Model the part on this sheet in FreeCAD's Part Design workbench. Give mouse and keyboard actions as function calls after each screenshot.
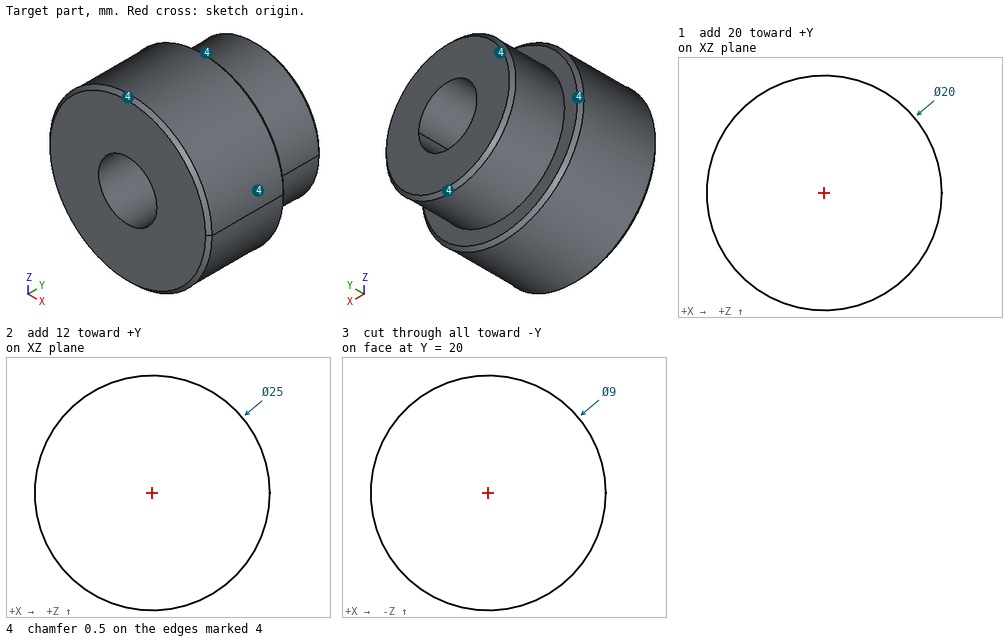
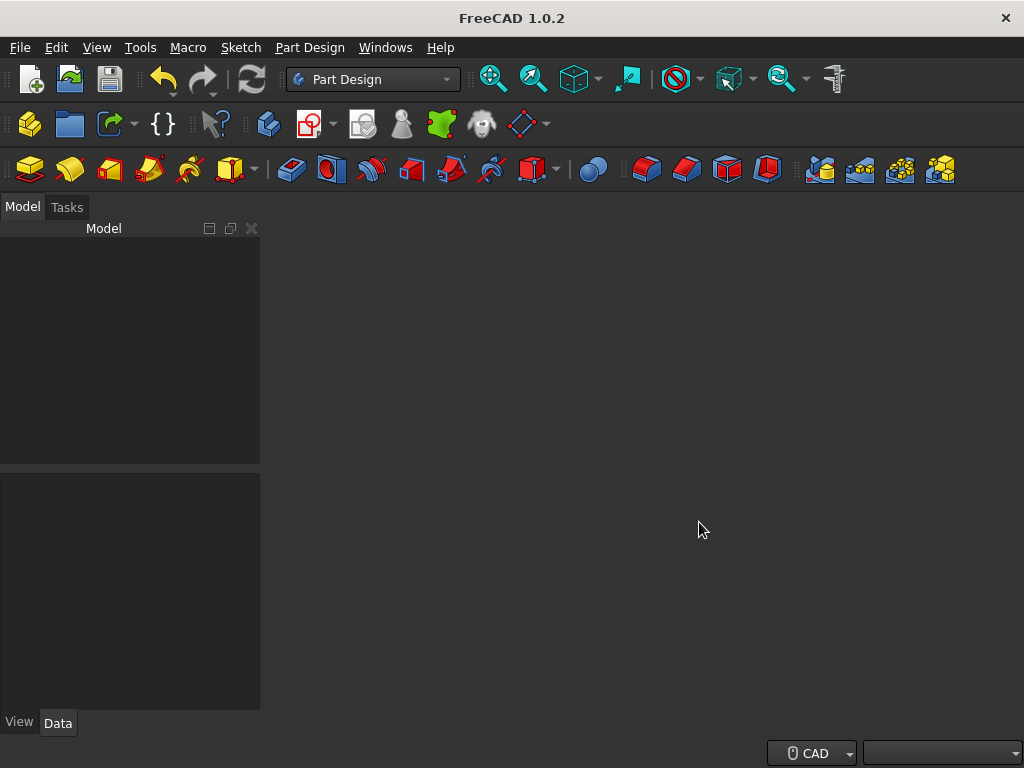
click(30, 80)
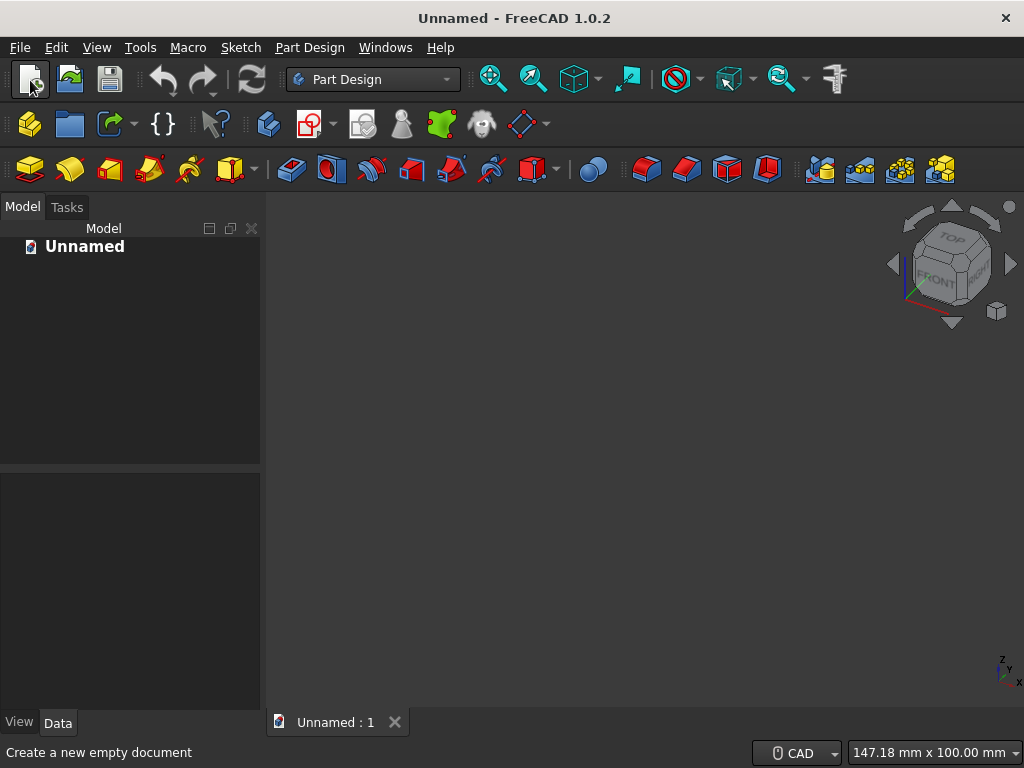
click(310, 124)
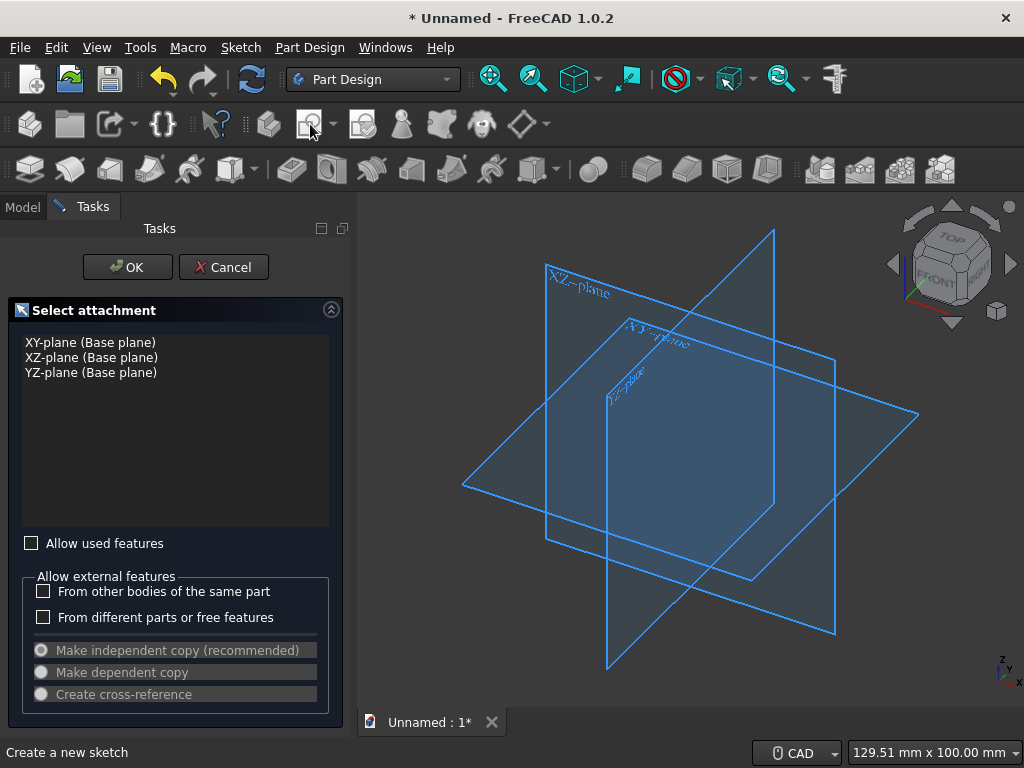
click(82, 358)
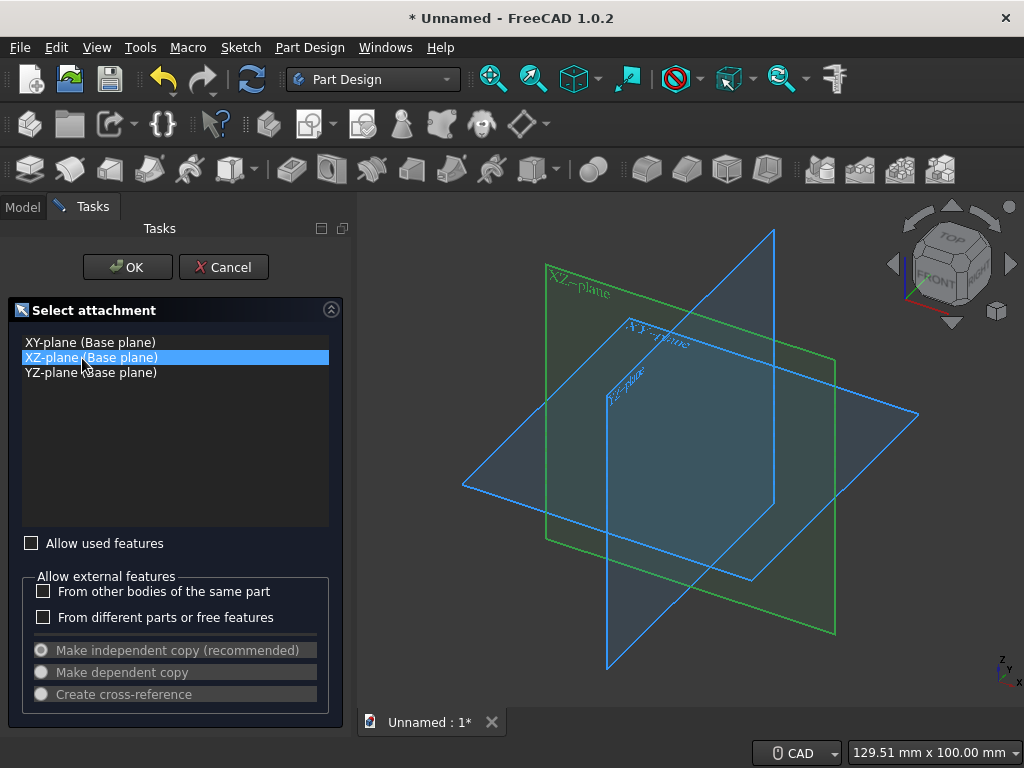
click(128, 267)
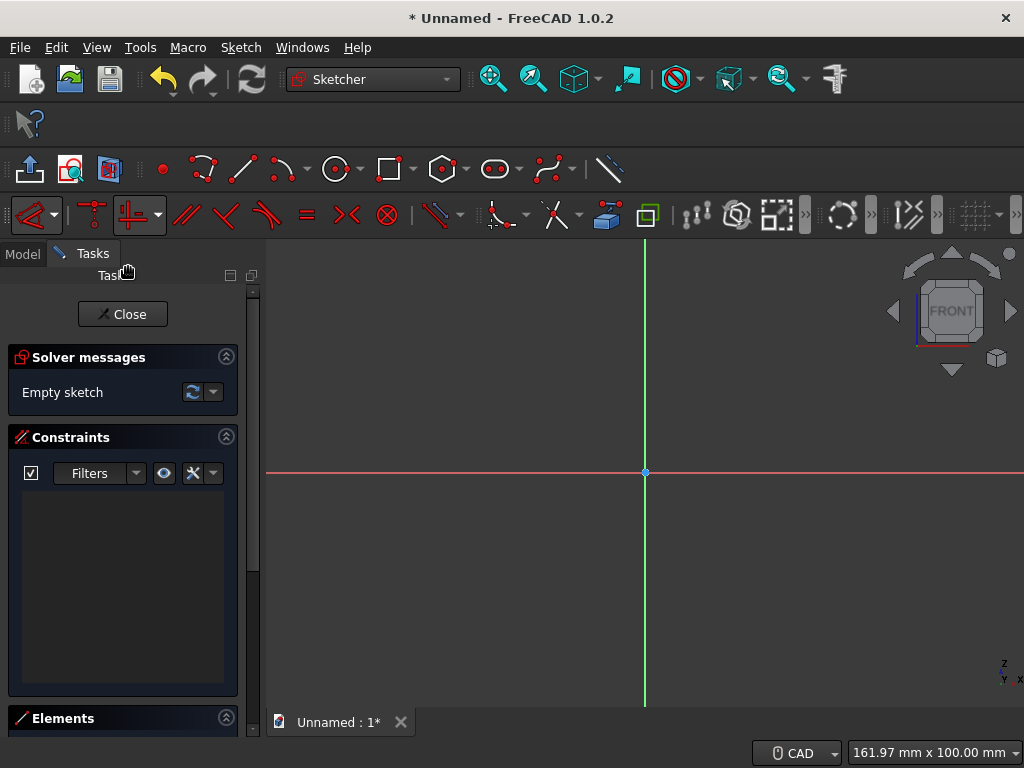
scroll(675, 473, up, 6)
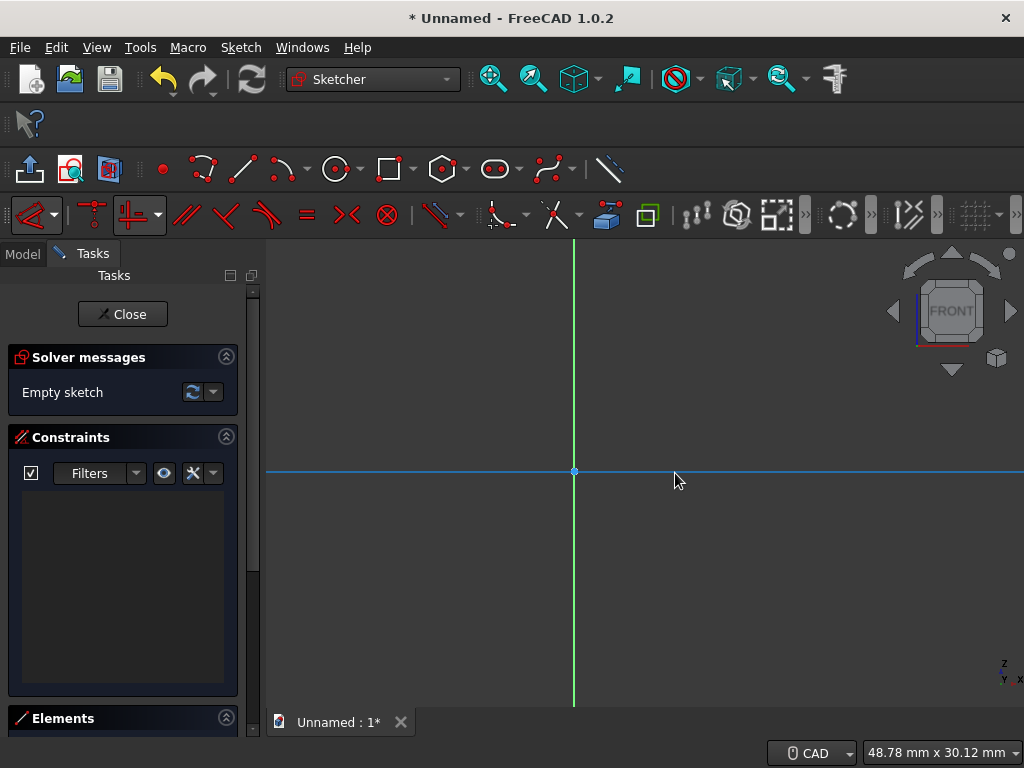
click(336, 170)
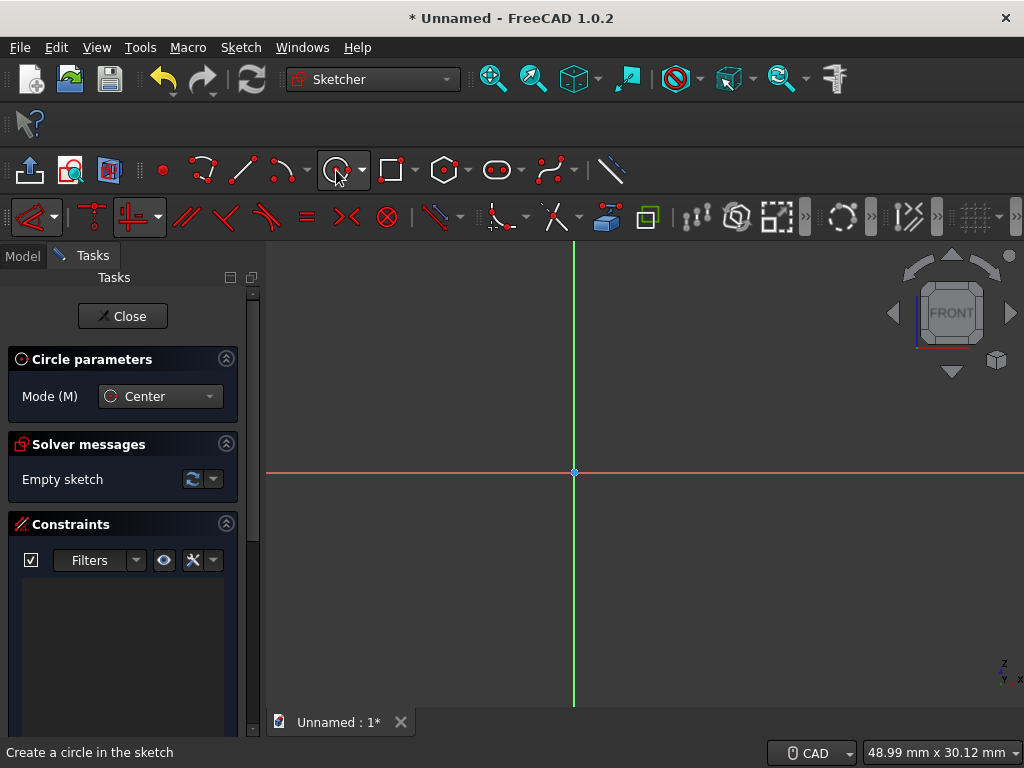
click(574, 473)
click(684, 363)
key(Escape)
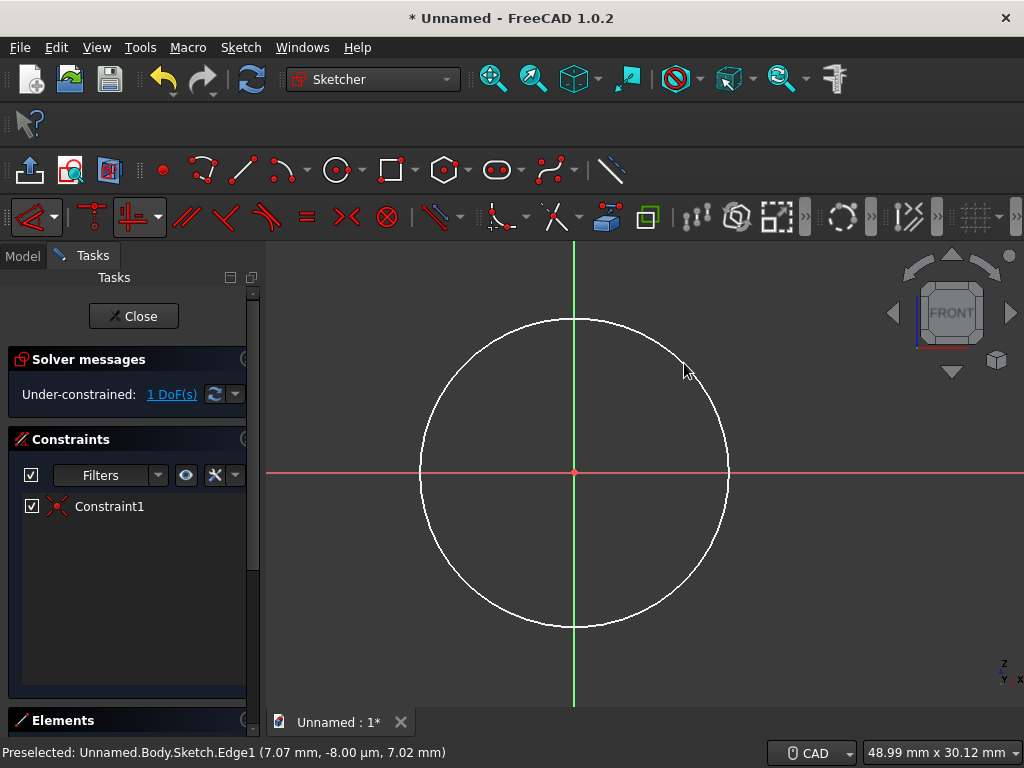
click(683, 363)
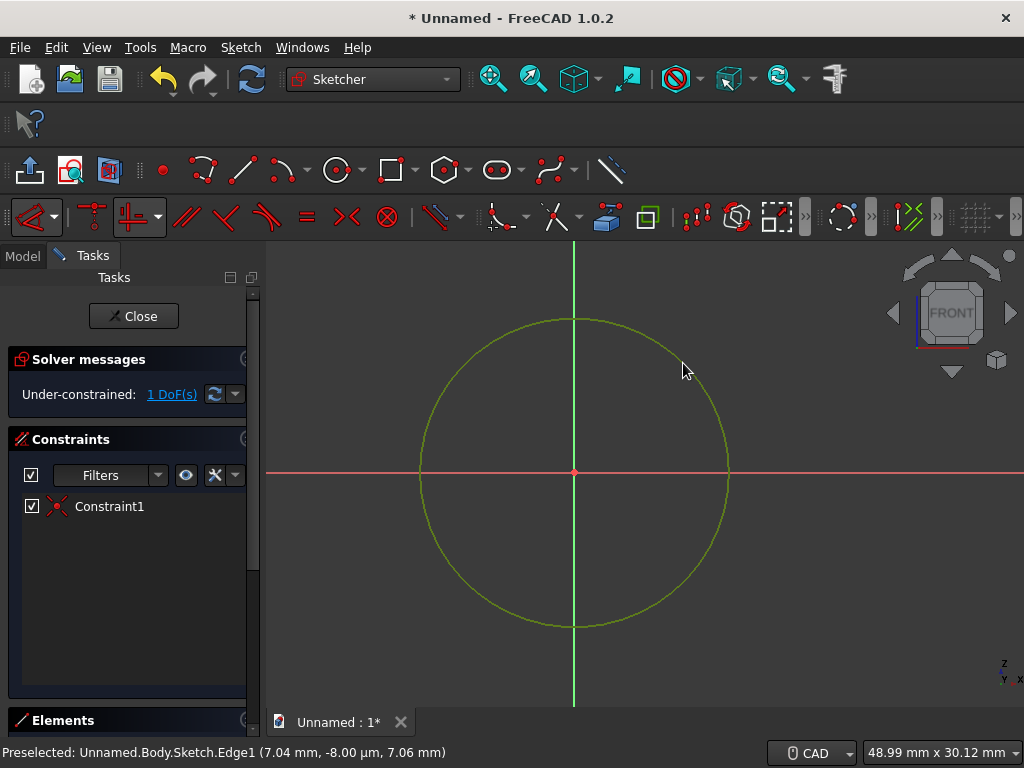
click(56, 218)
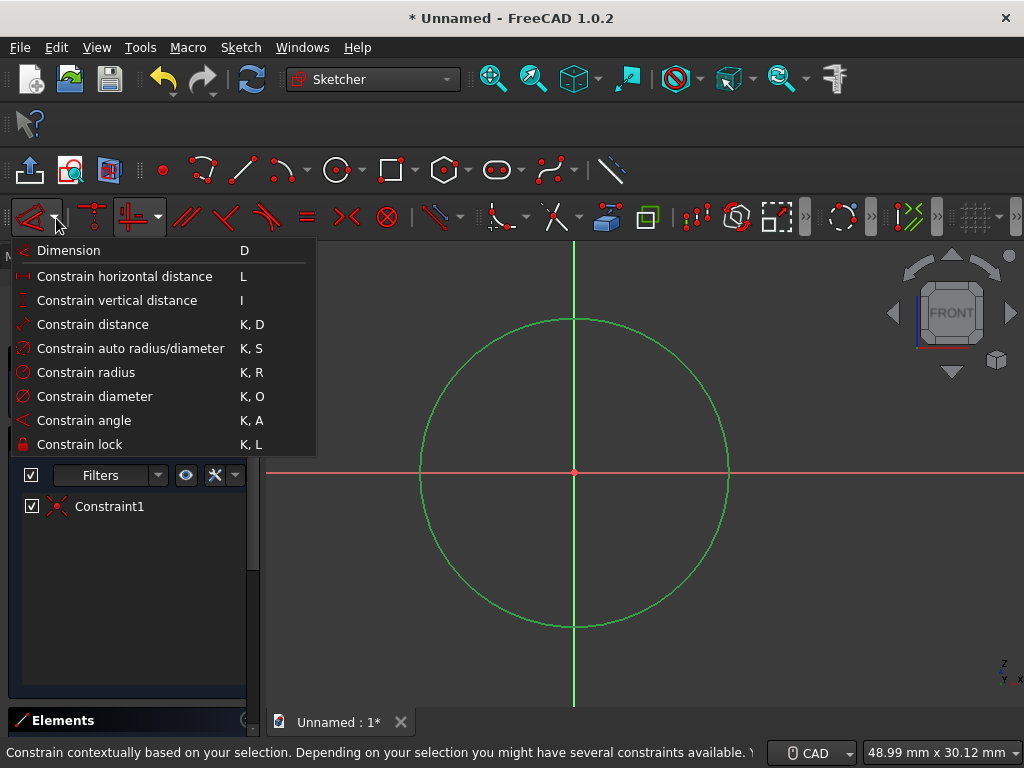
click(164, 396)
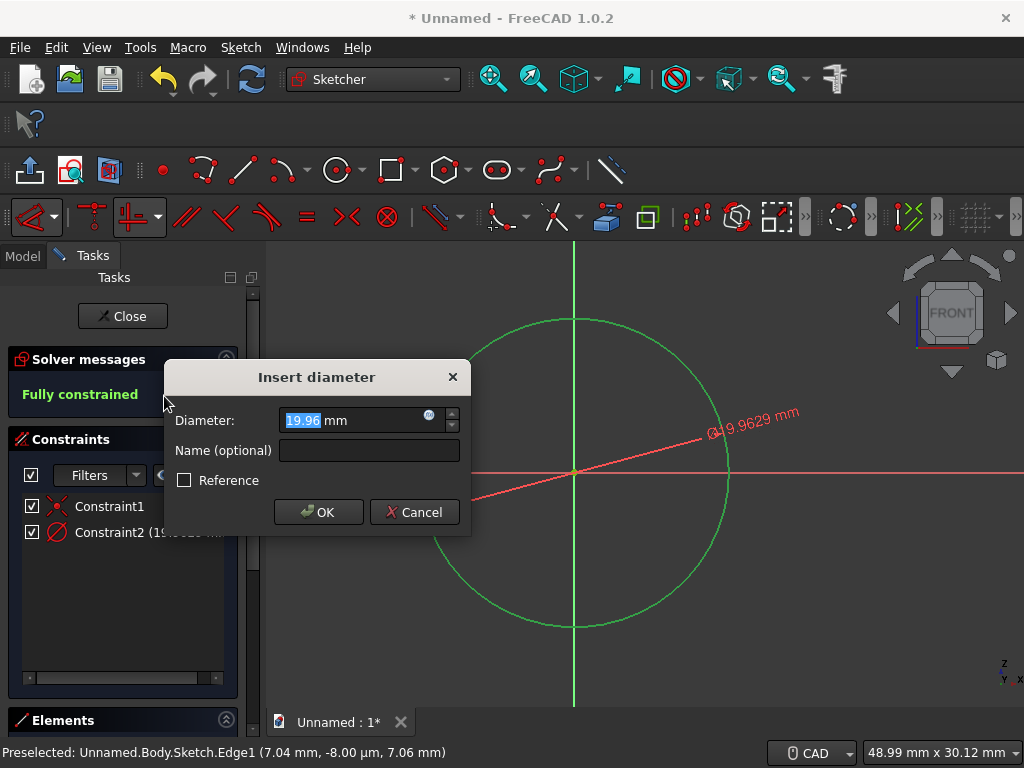
text(20)
key(Return)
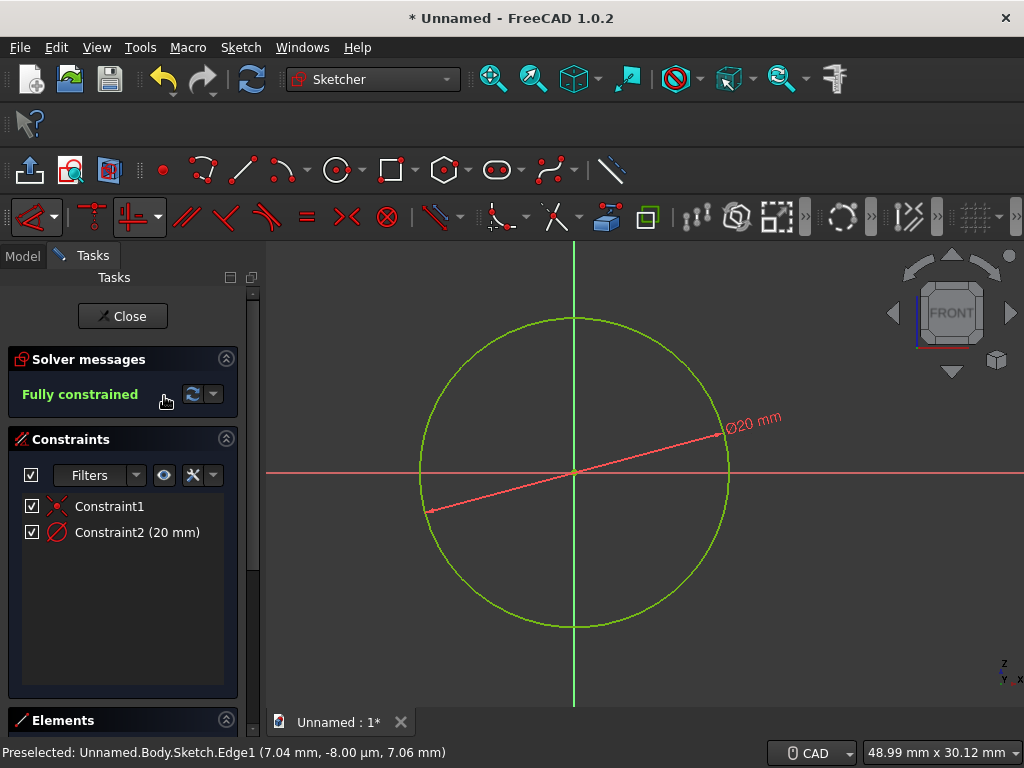
click(123, 316)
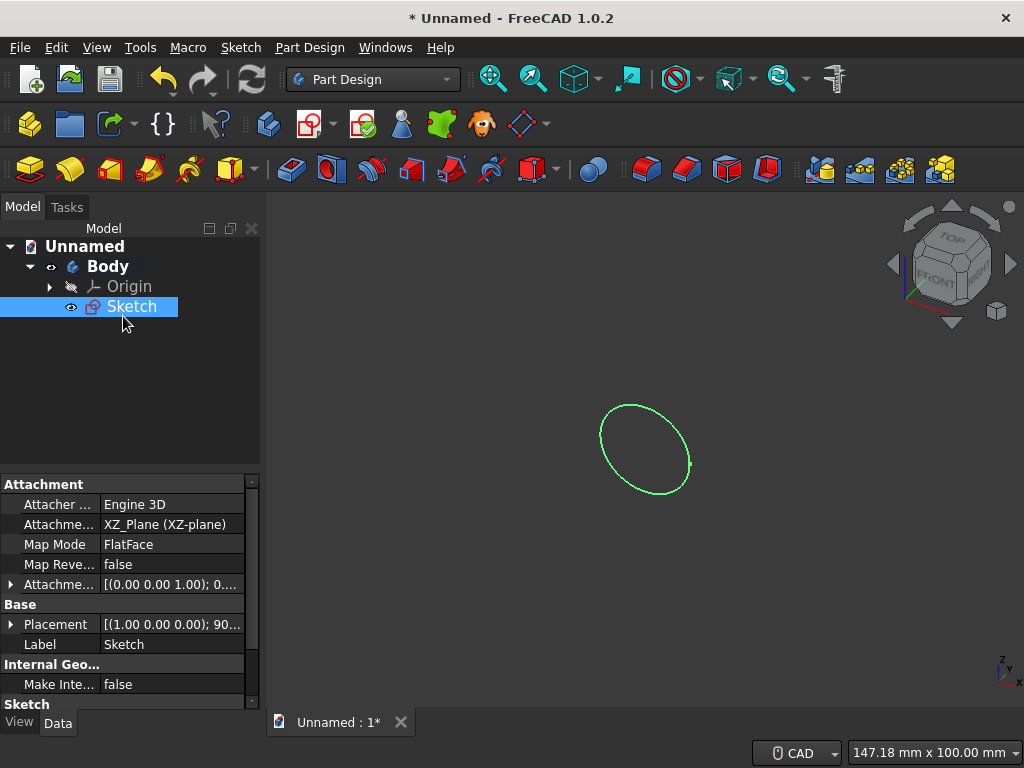
click(30, 170)